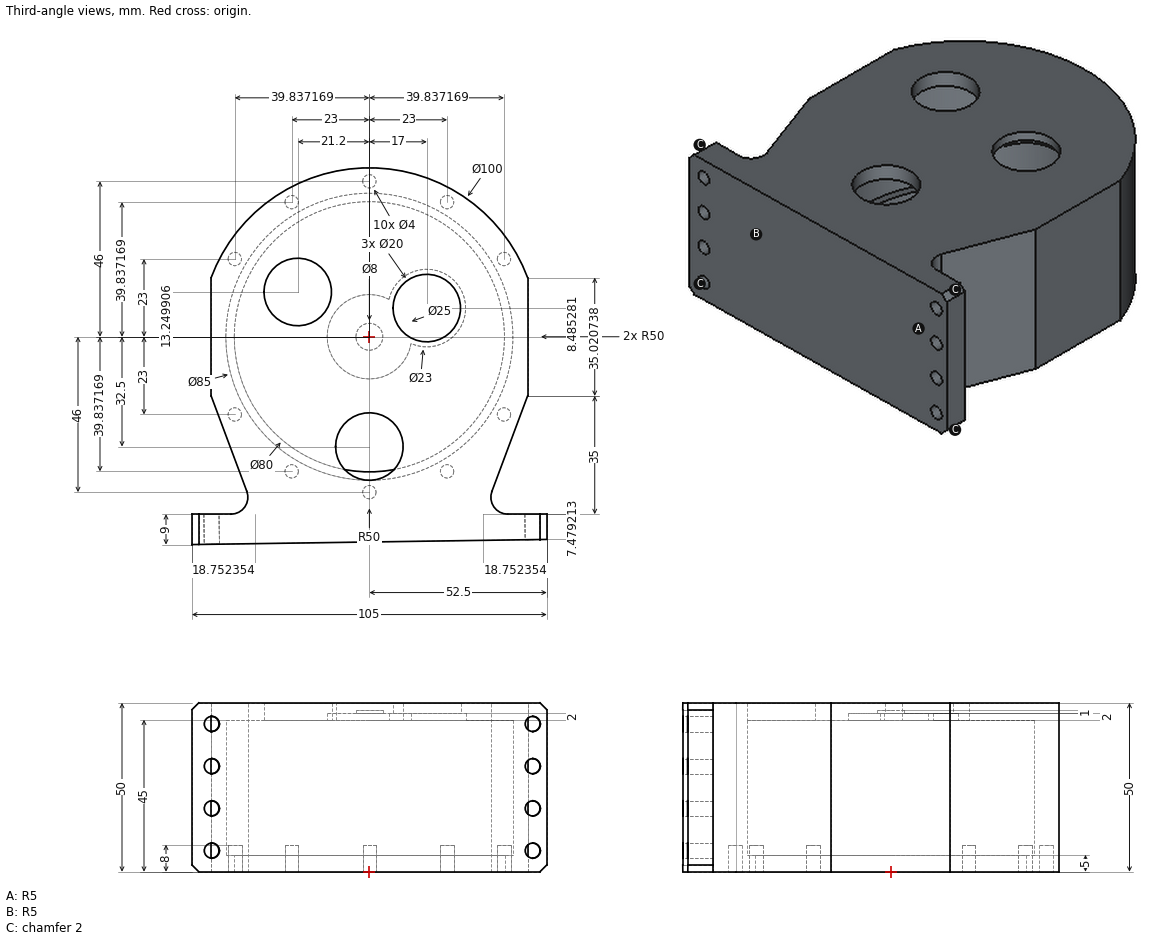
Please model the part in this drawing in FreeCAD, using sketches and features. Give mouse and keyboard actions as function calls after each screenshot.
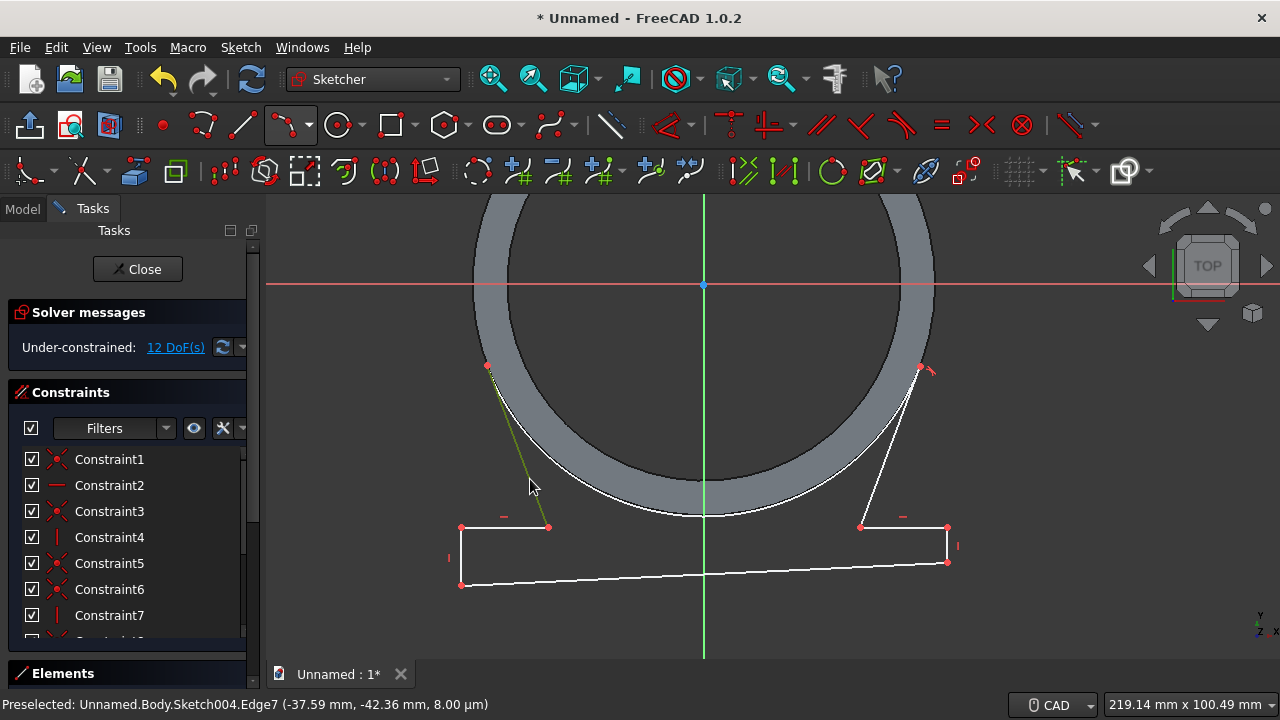
click(596, 490)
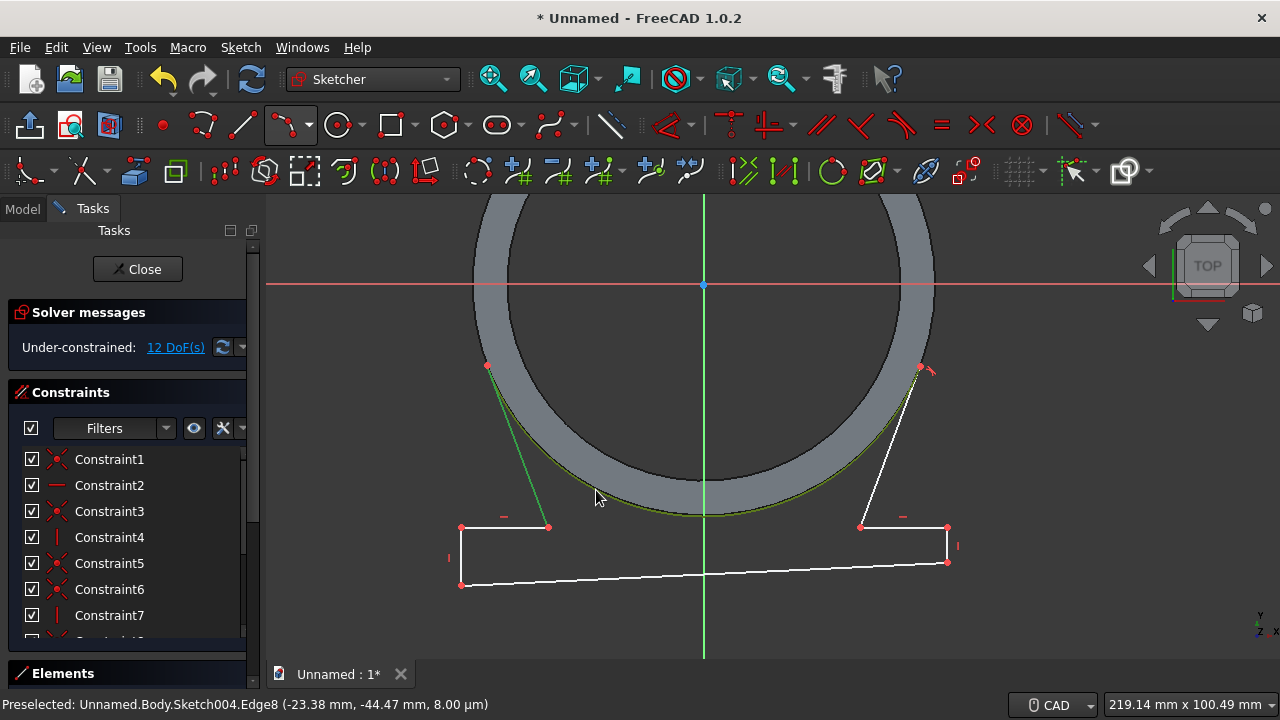
click(902, 126)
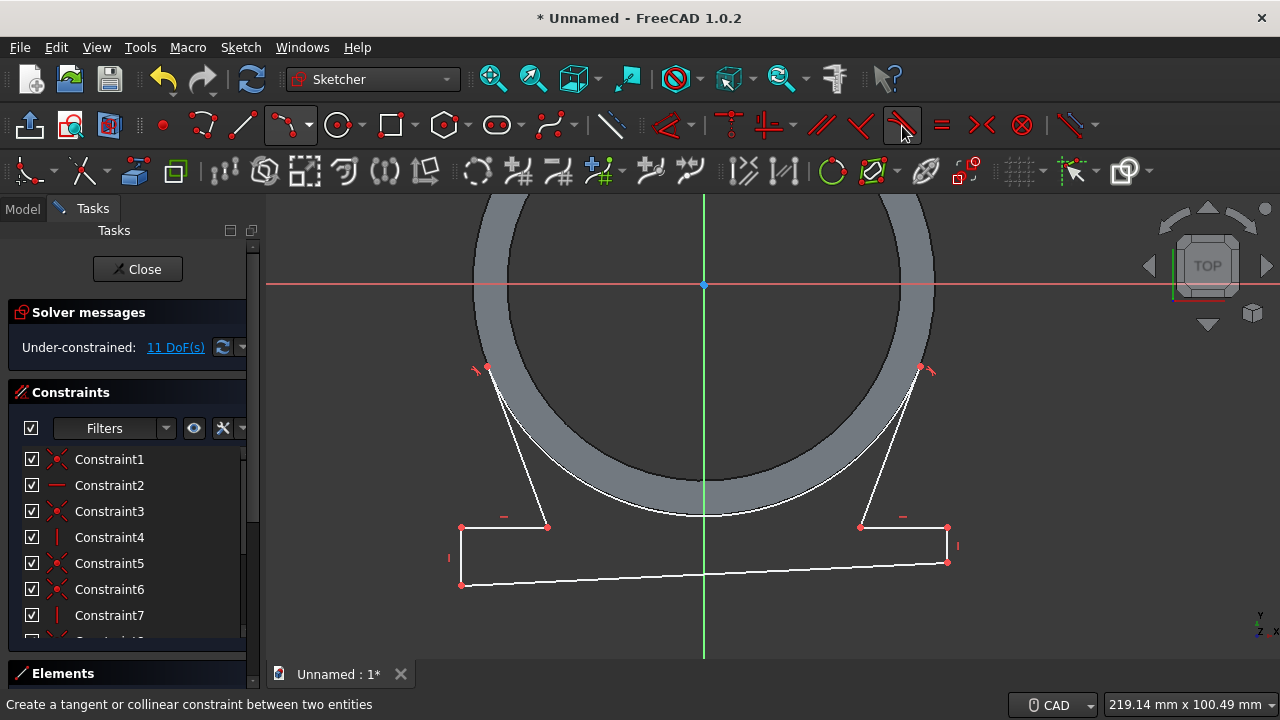
drag(694, 274, 714, 295)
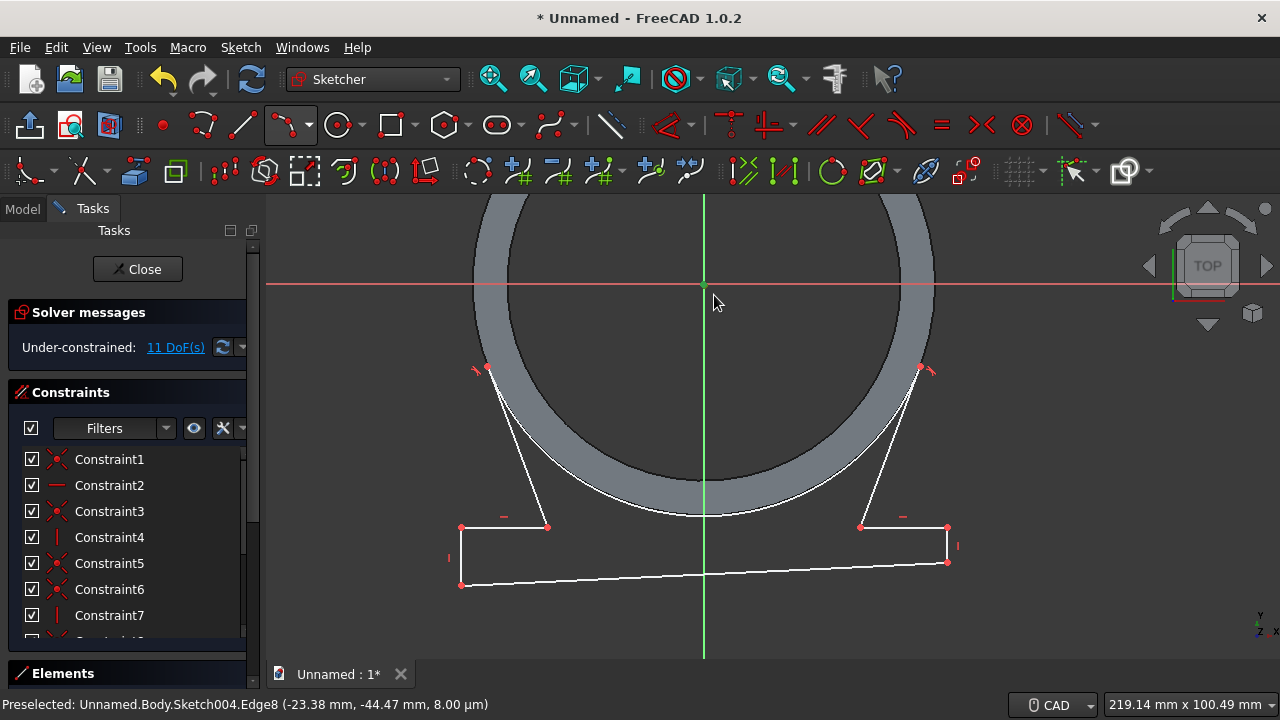
key(c)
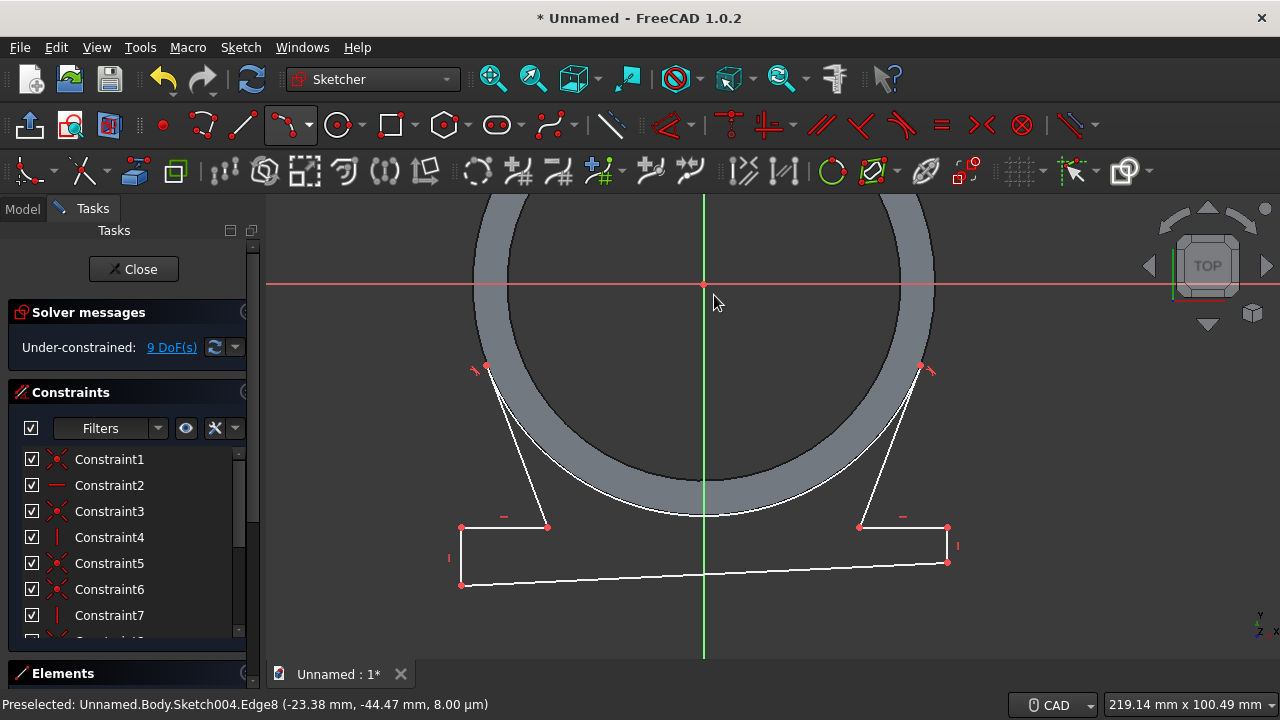
click(666, 126)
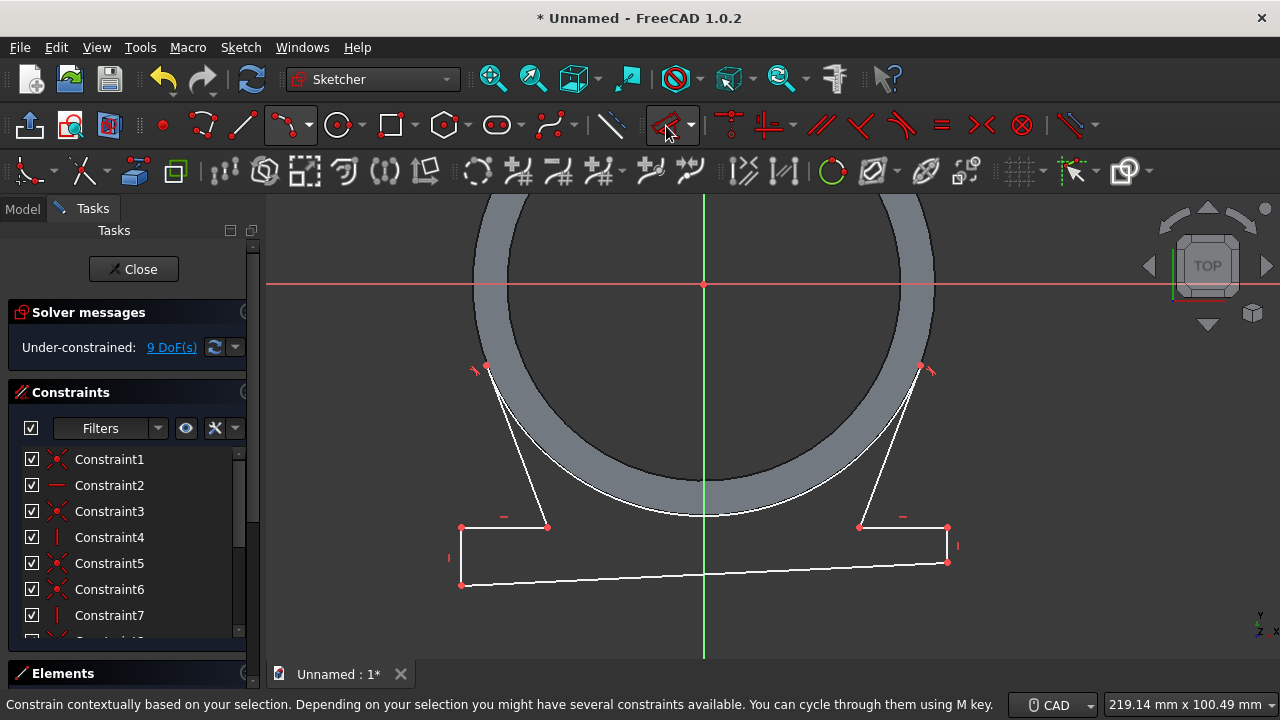
click(596, 489)
click(581, 517)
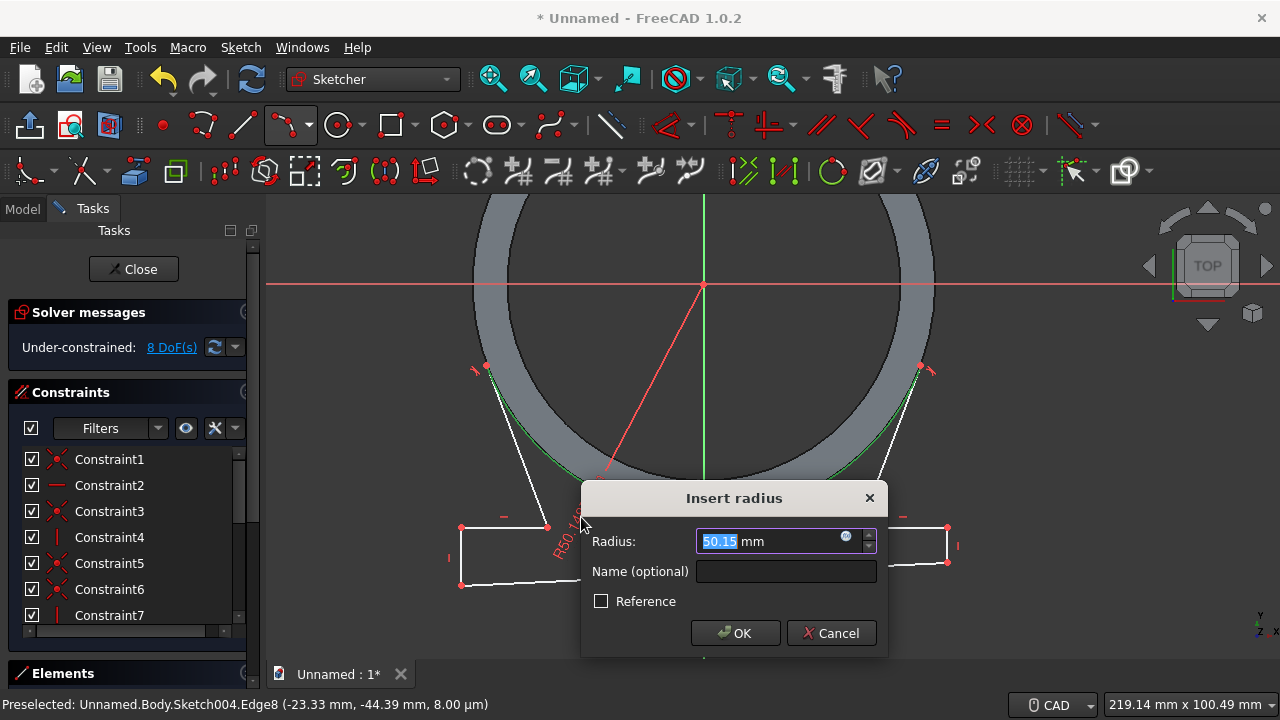
text(50)
key(Return)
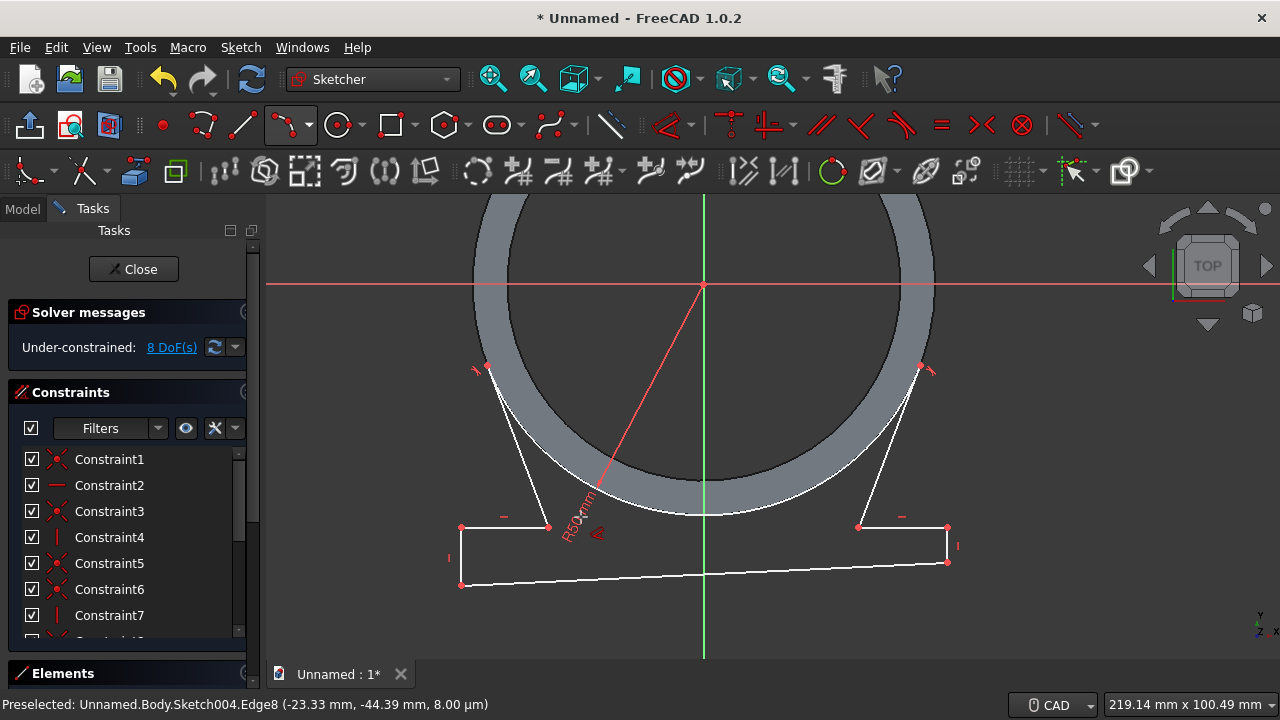
click(461, 569)
click(427, 557)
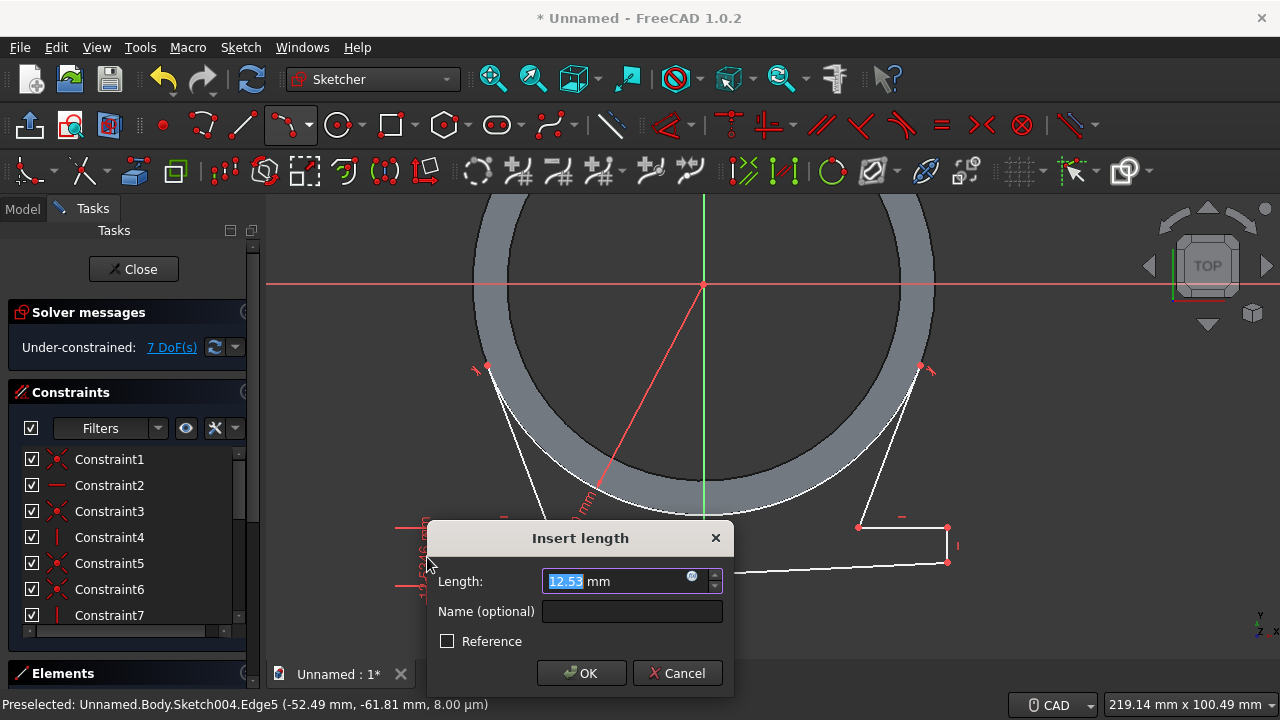
text(9)
key(Return)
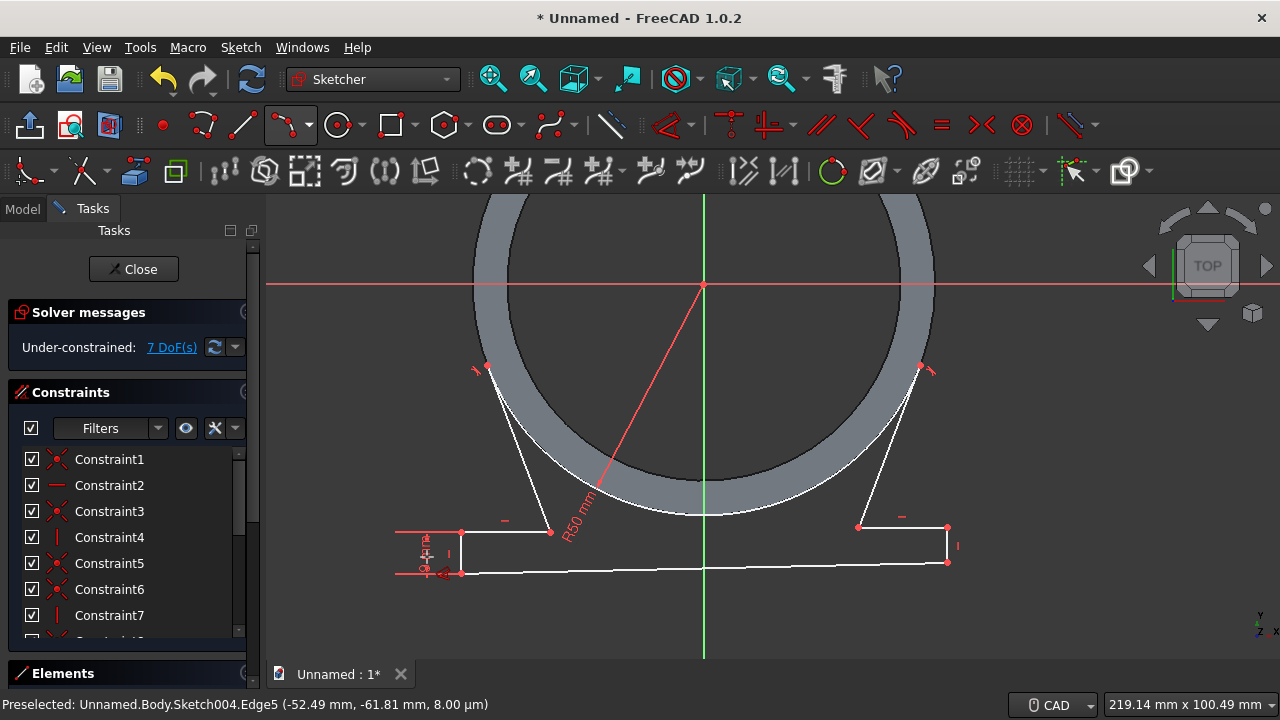
click(877, 479)
click(954, 447)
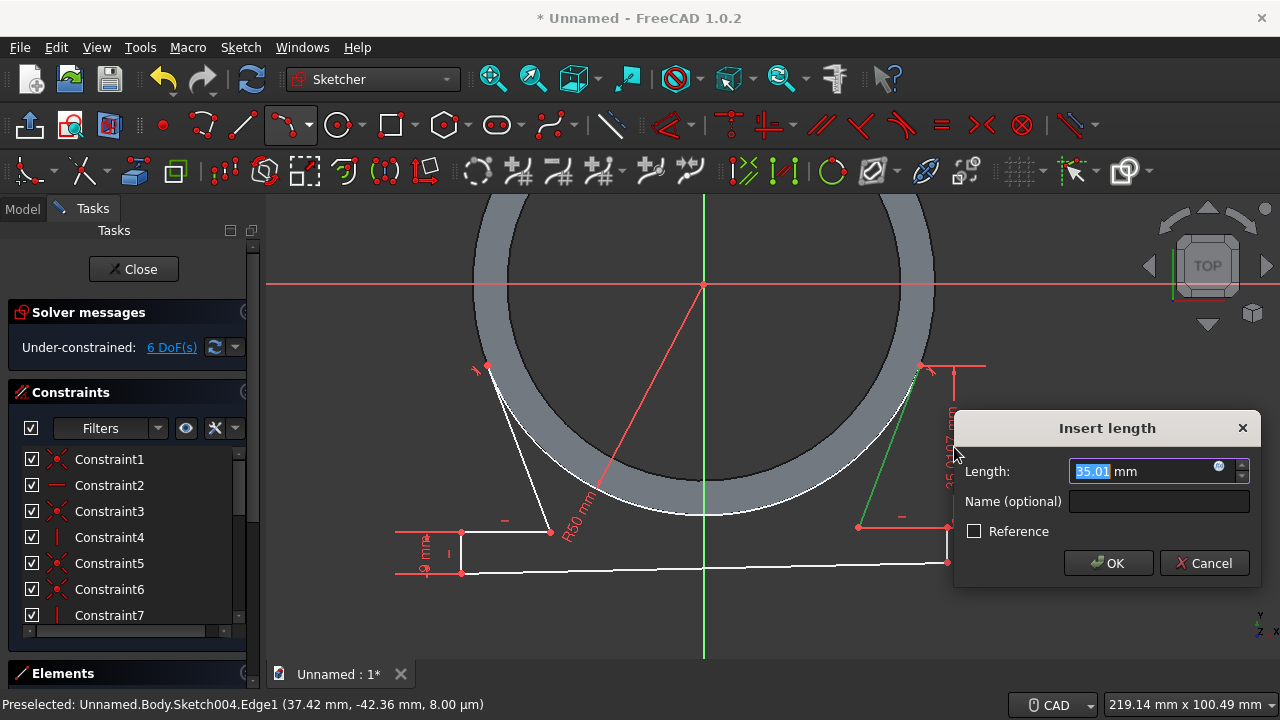
text(35)
key(Return)